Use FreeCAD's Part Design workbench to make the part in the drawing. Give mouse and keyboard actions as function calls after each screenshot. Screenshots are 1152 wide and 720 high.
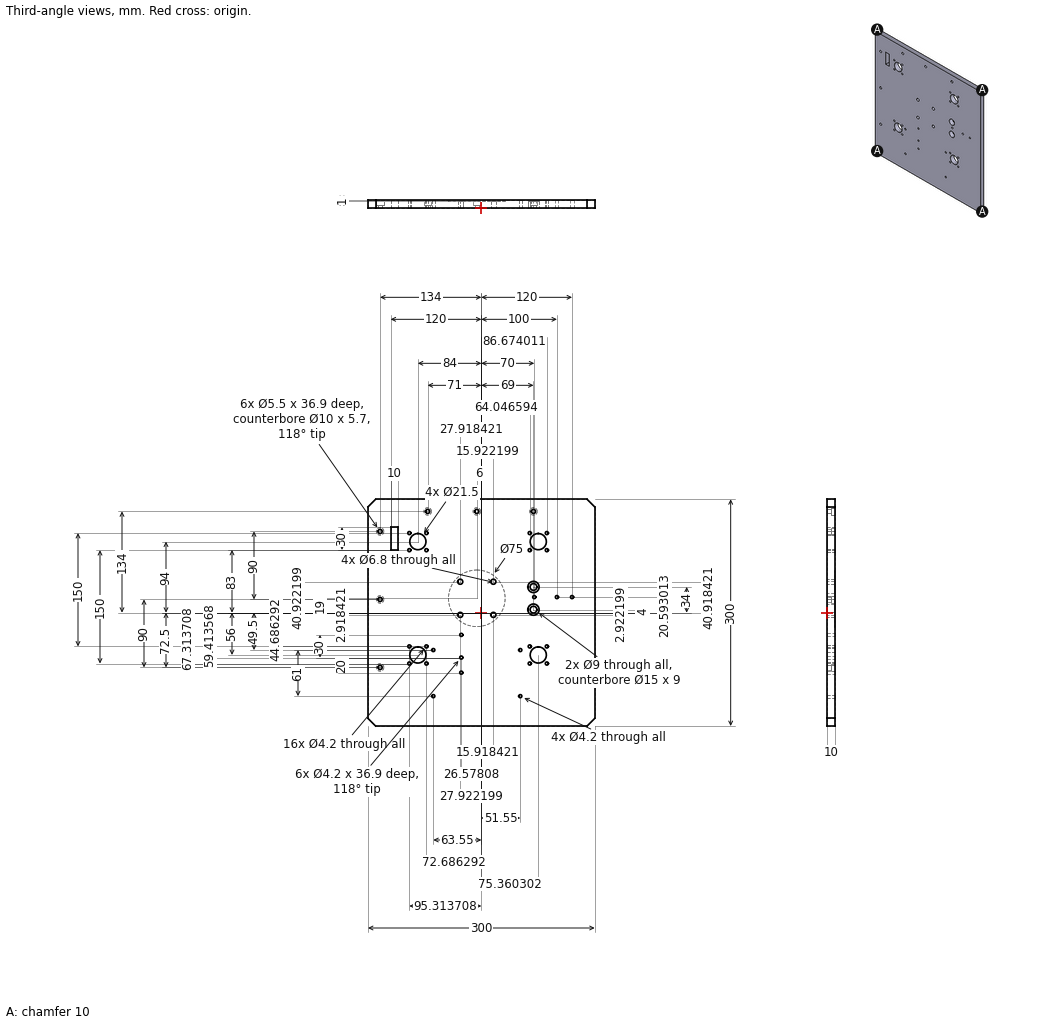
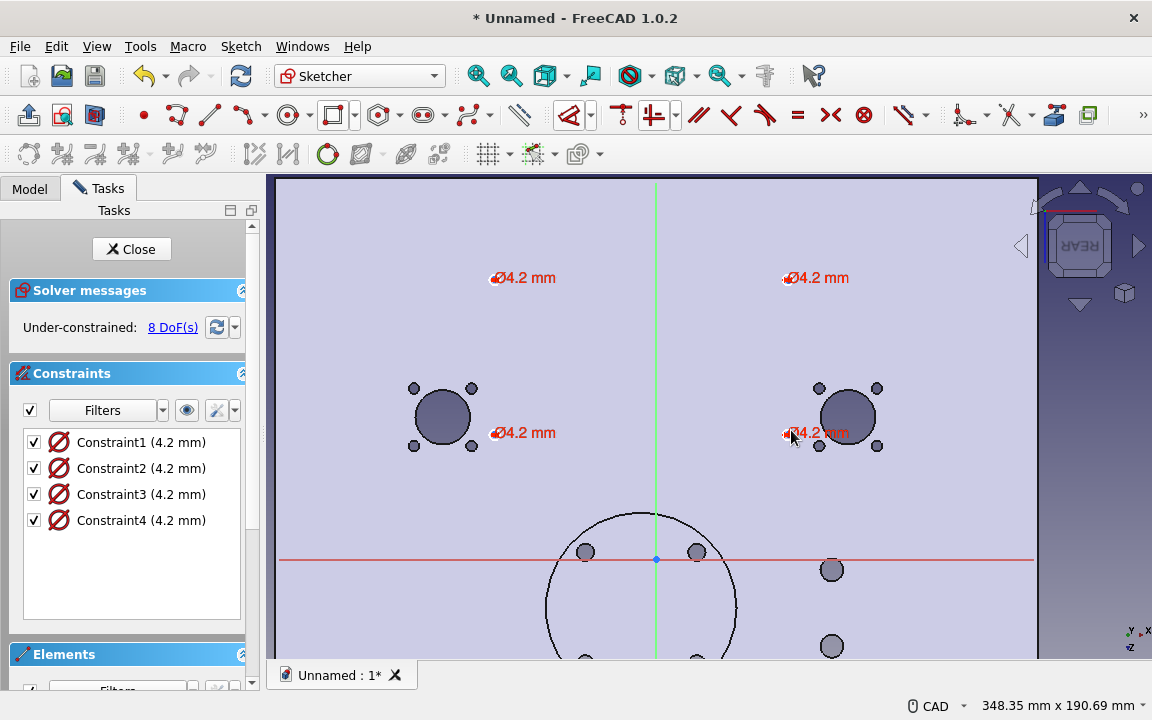
click(788, 280)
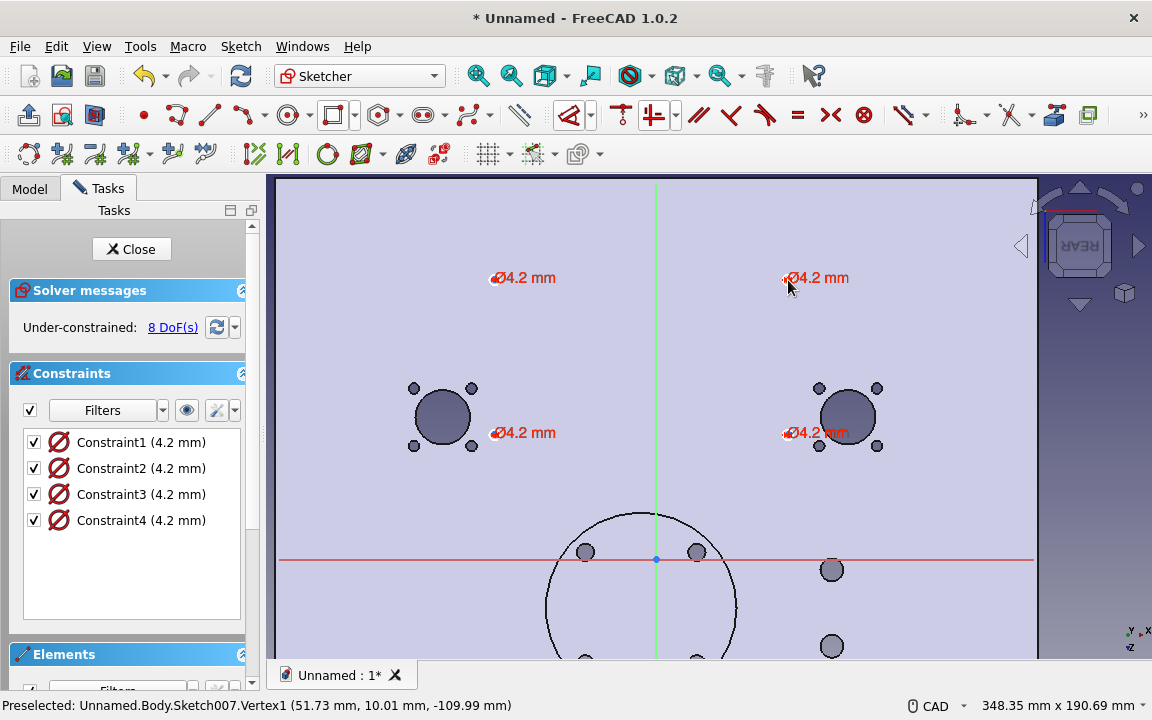
click(495, 280)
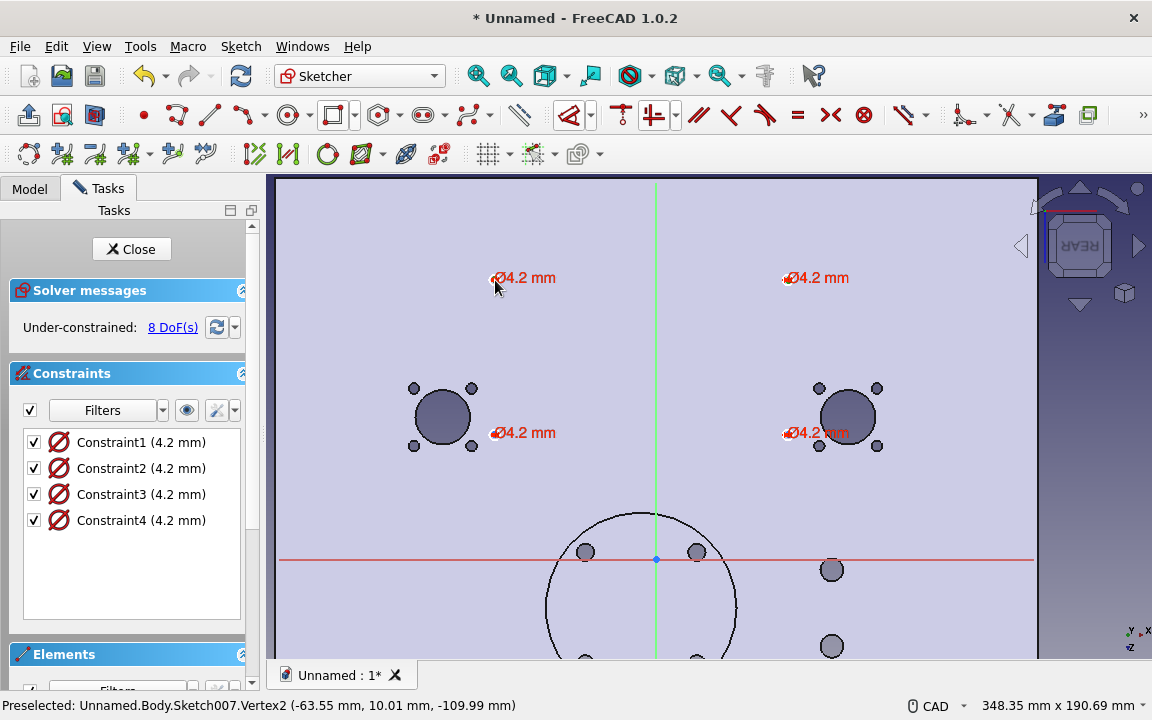
click(676, 116)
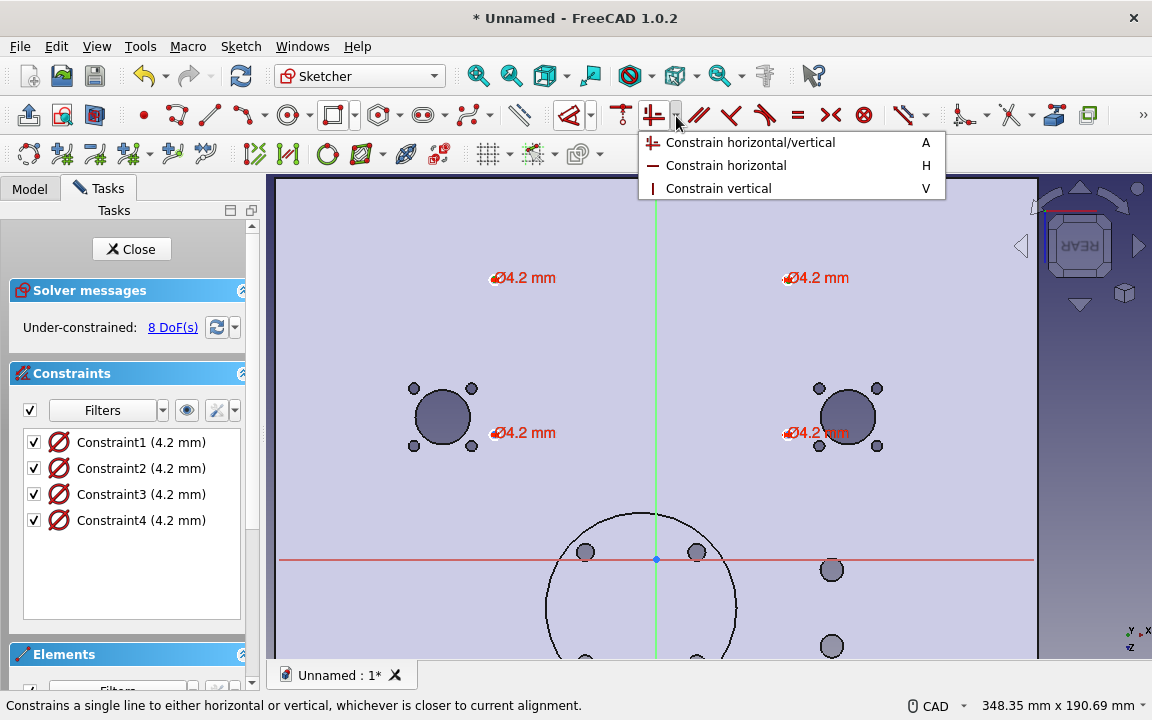
click(792, 166)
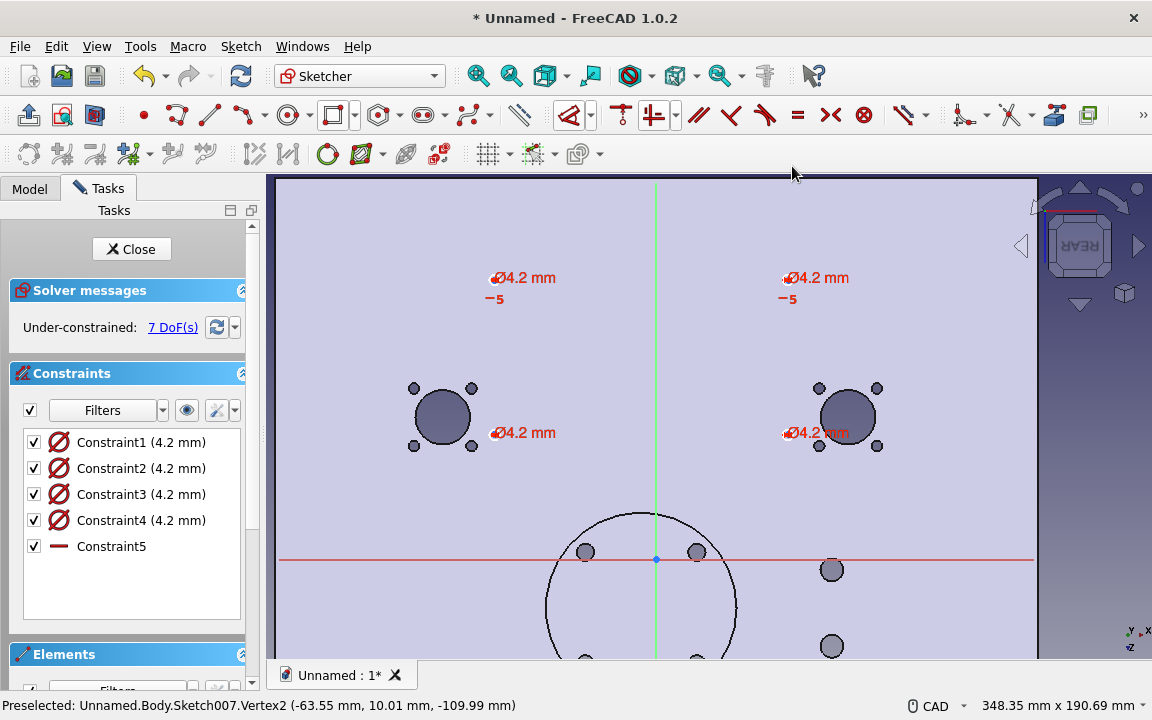
click(495, 280)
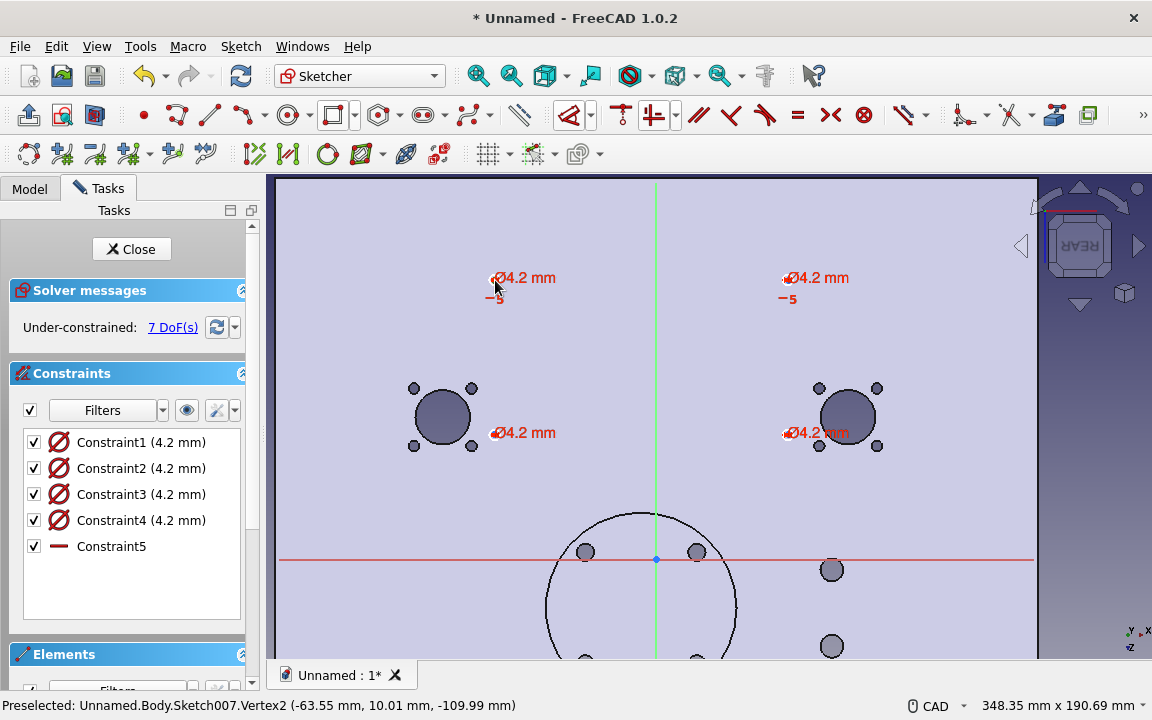
click(495, 435)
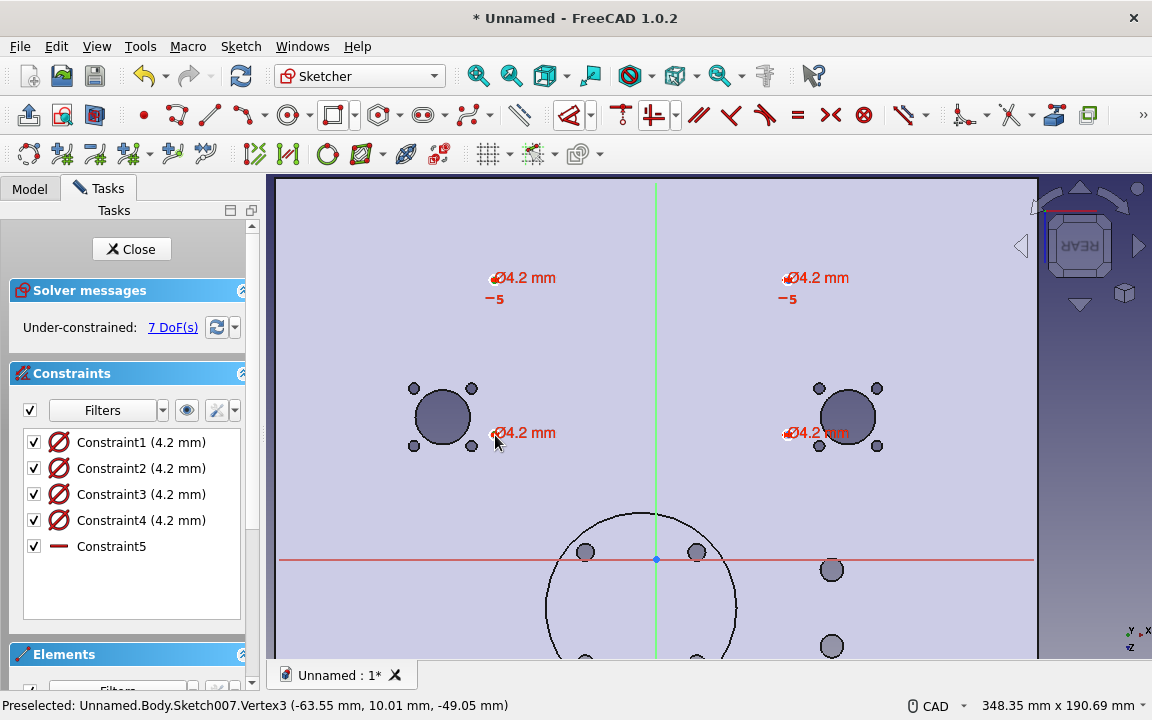
click(676, 116)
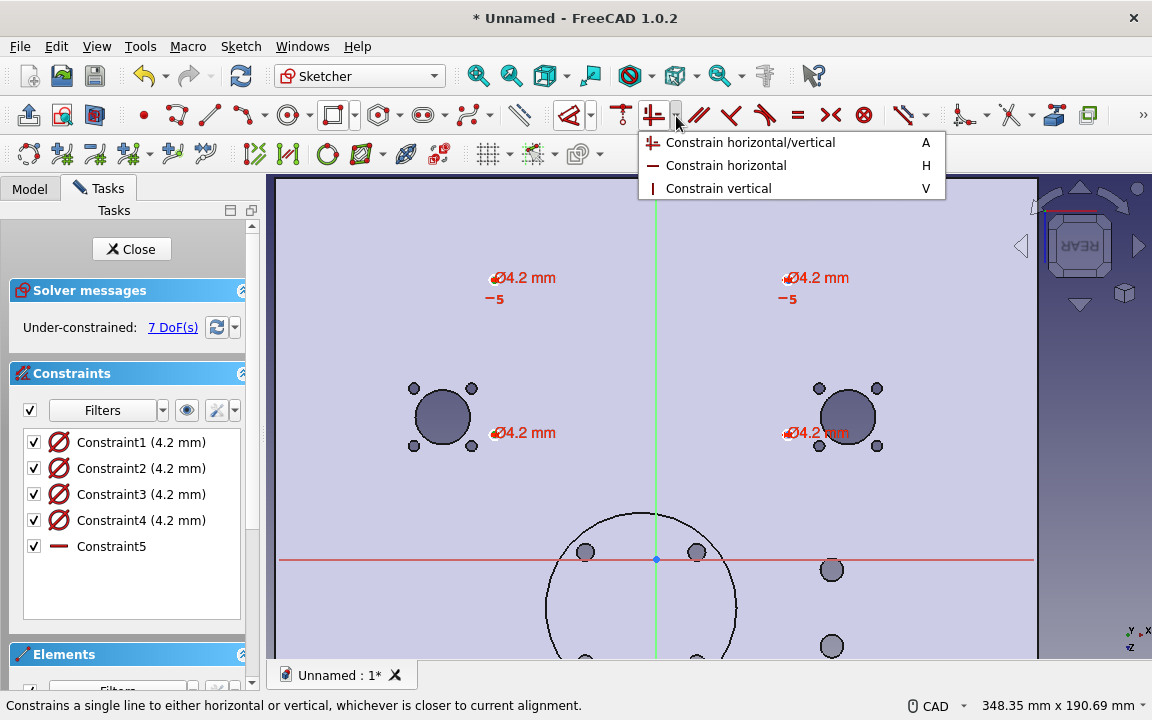
click(792, 188)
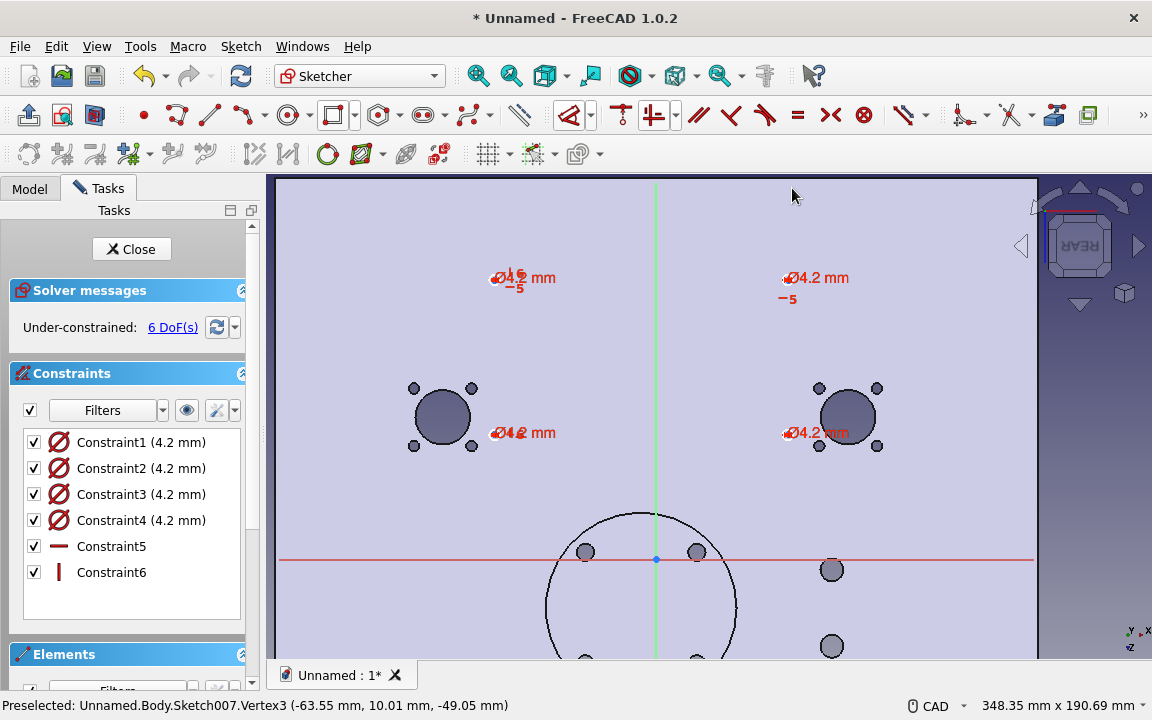
click(788, 280)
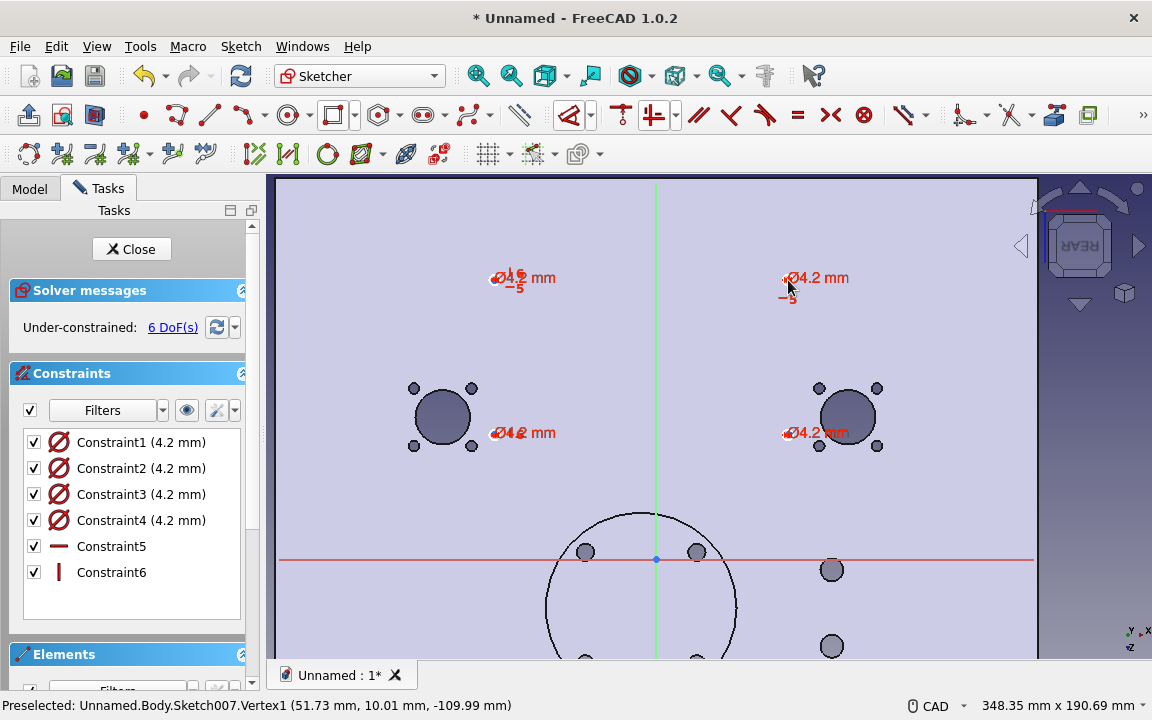
click(788, 435)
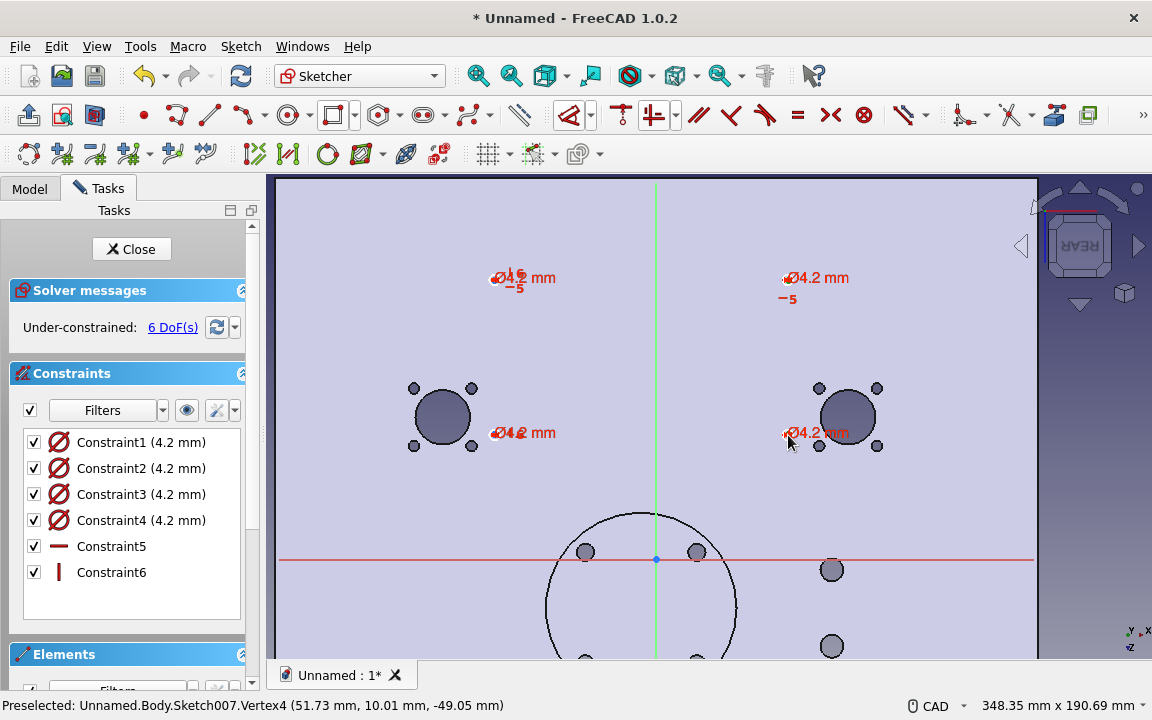
click(676, 116)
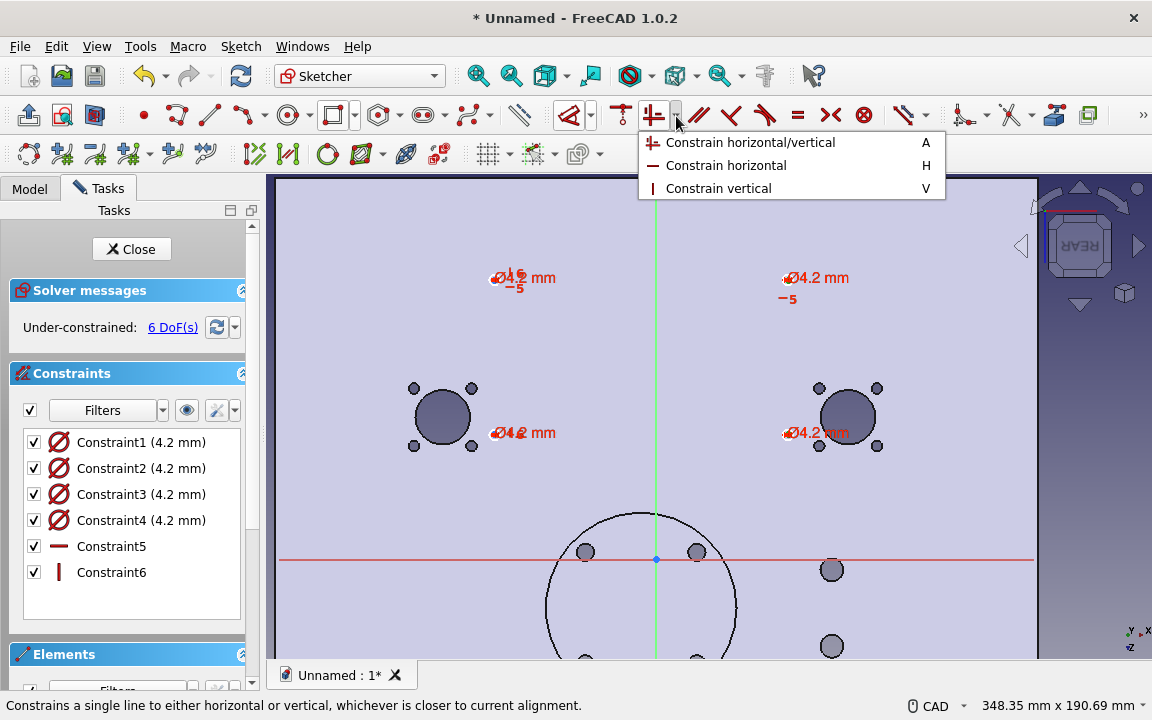
click(792, 188)